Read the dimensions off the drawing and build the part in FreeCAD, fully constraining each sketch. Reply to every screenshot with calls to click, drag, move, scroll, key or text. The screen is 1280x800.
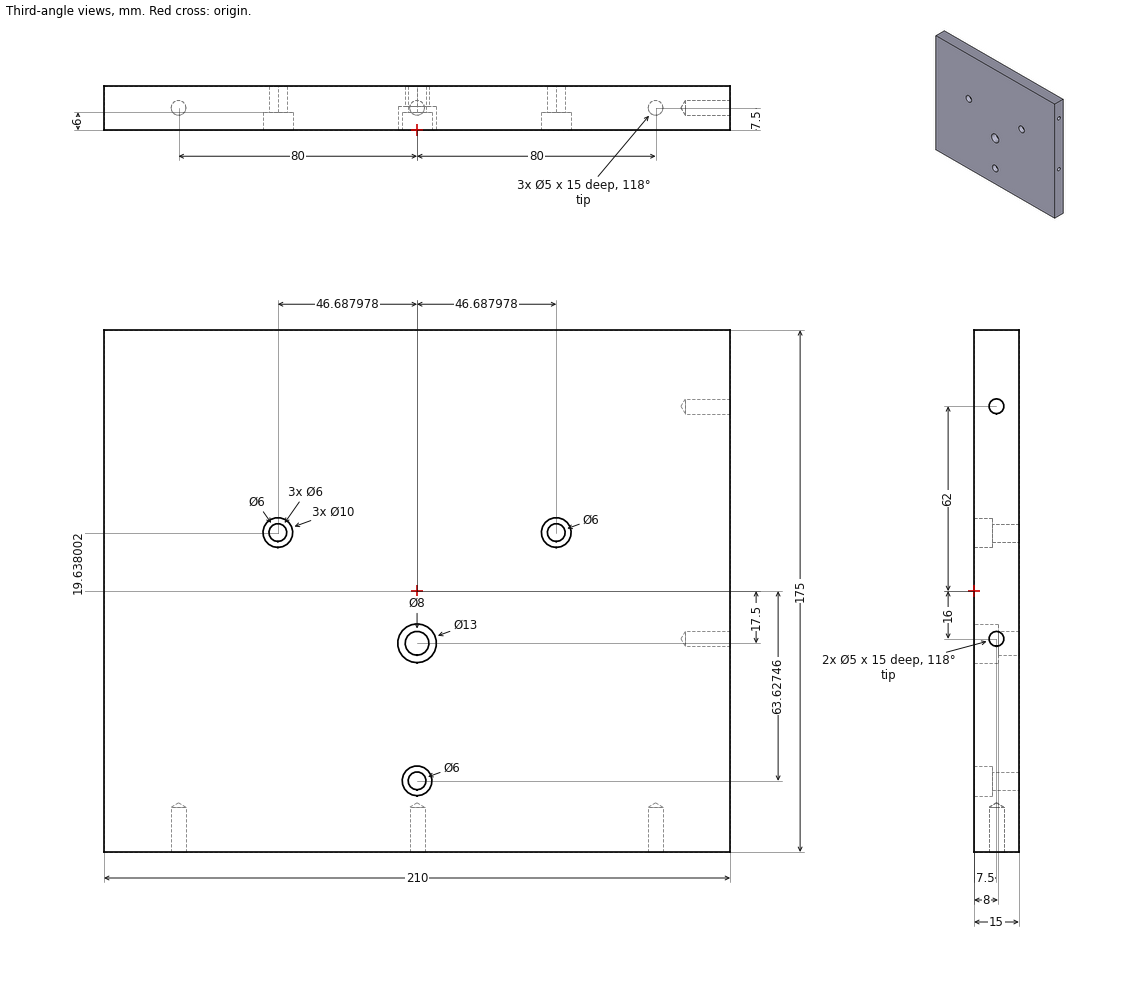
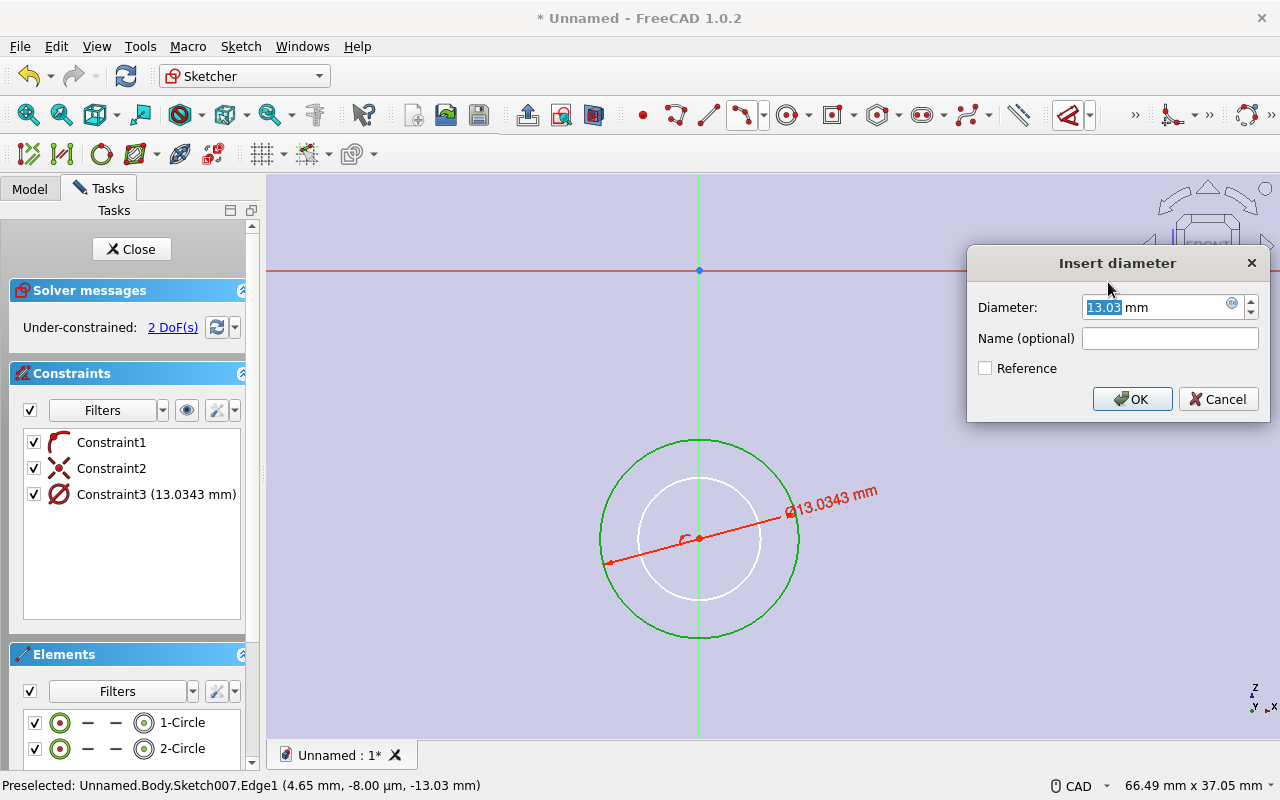
text(13)
key(Return)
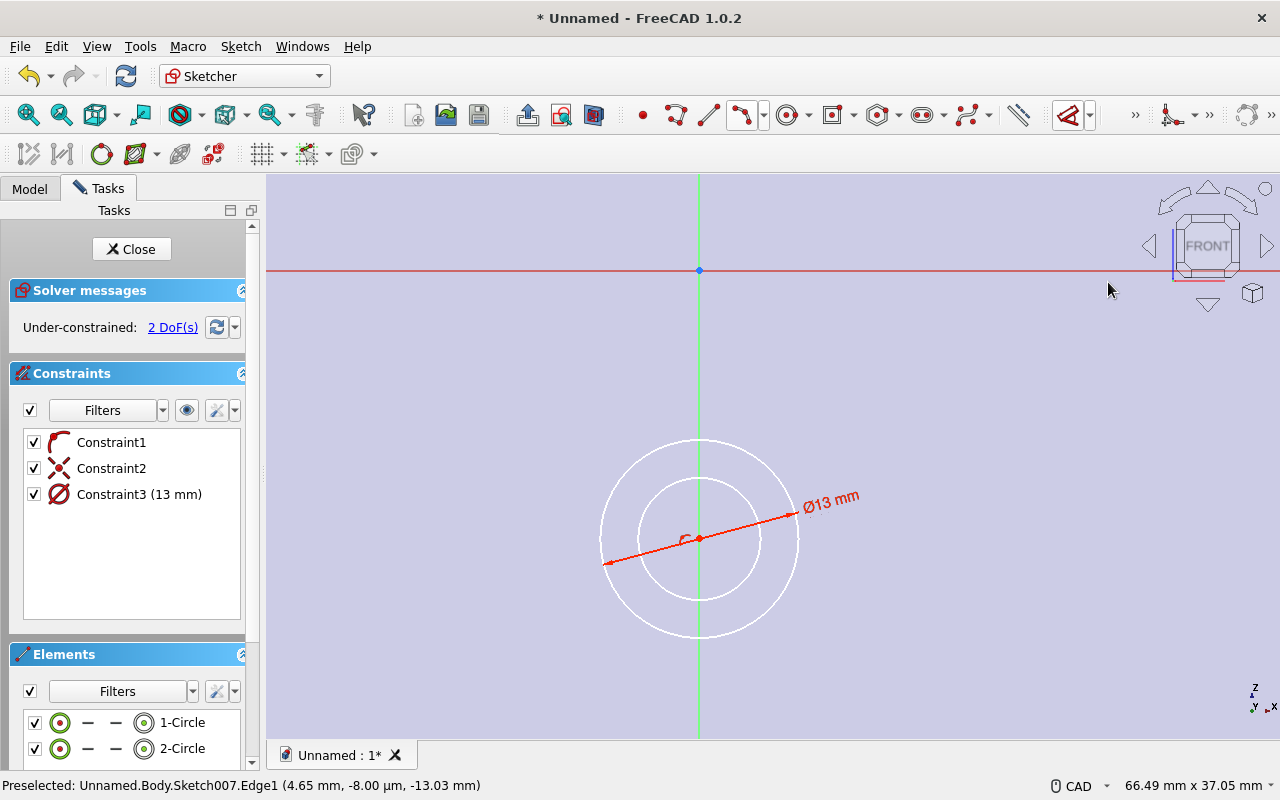
click(743, 496)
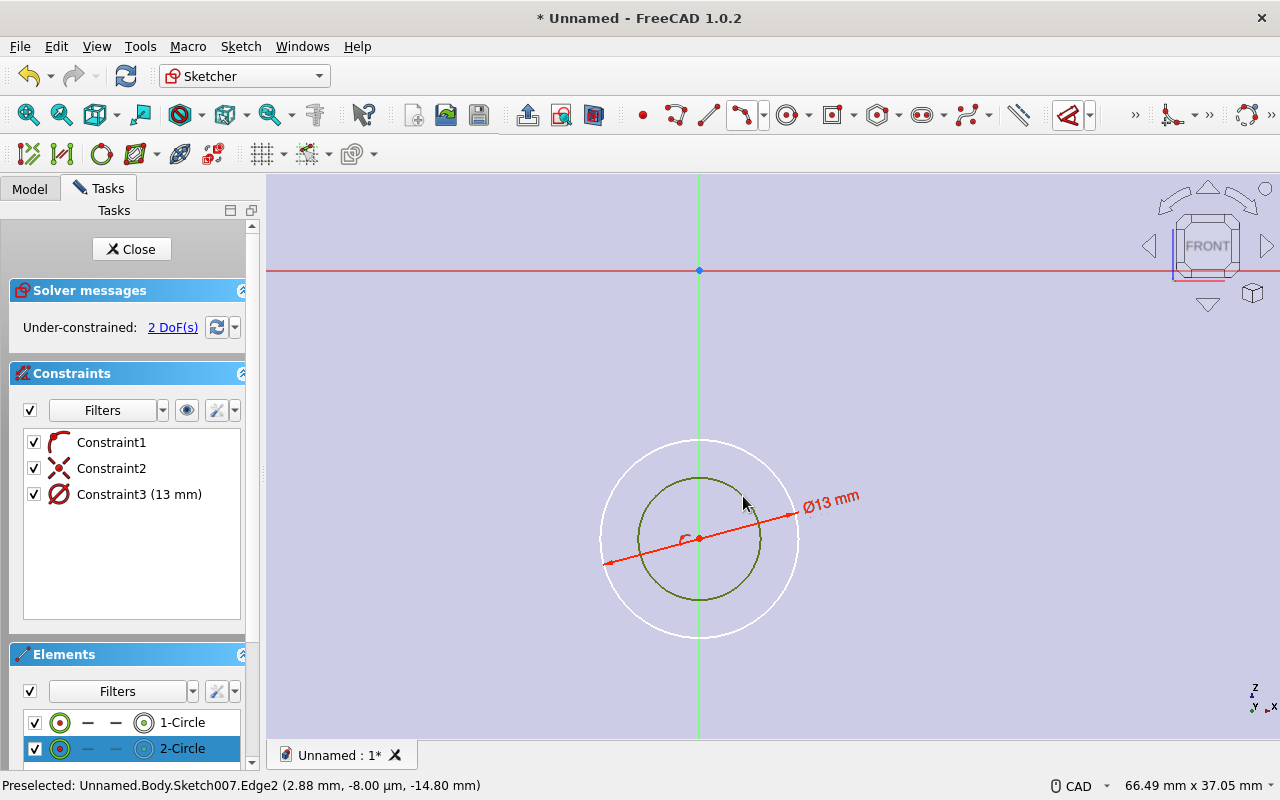
click(1090, 116)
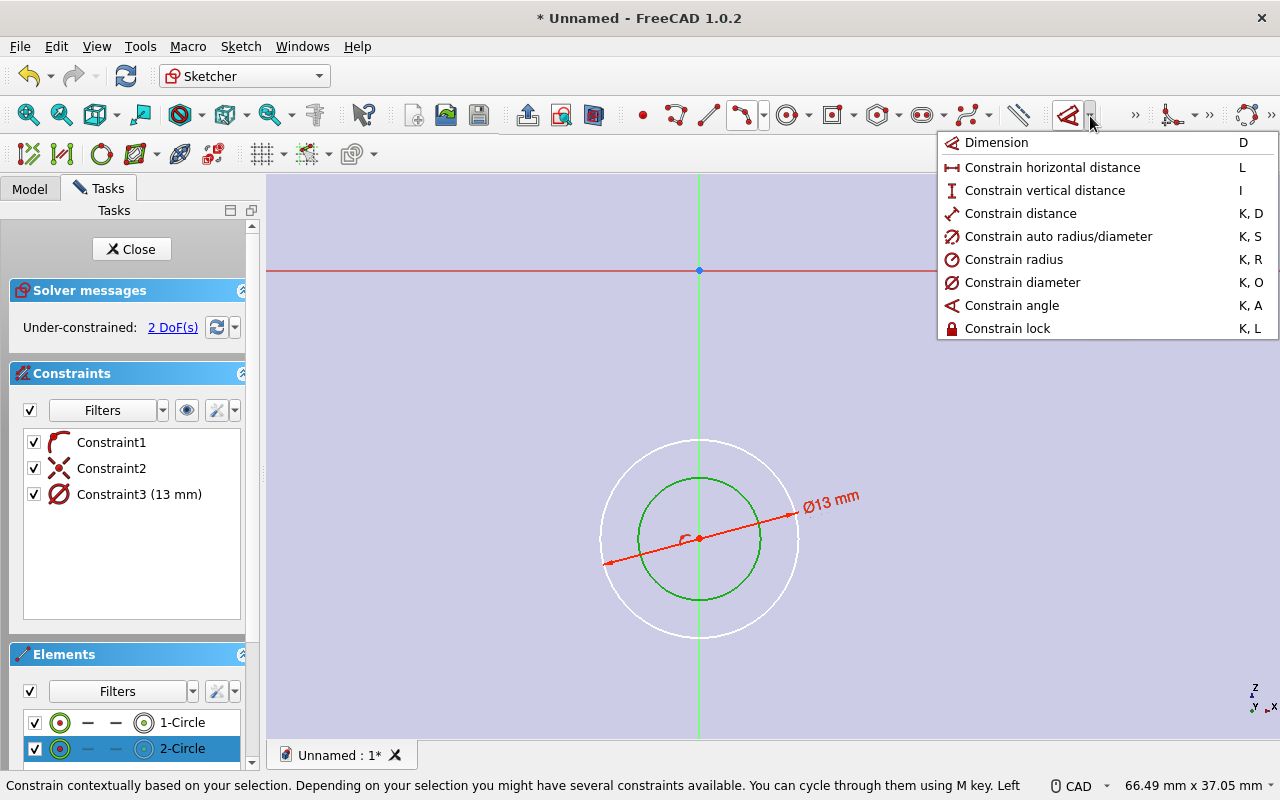
click(1108, 282)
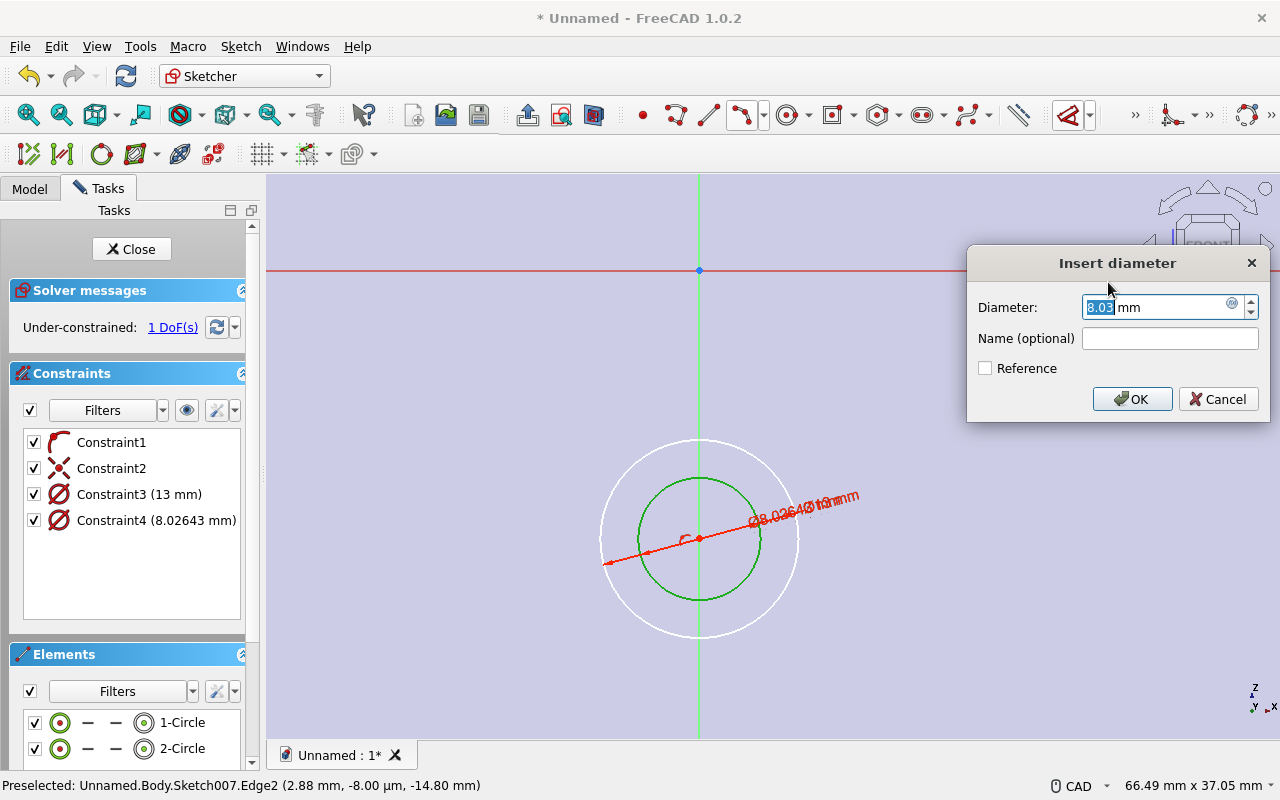
text(8)
key(Return)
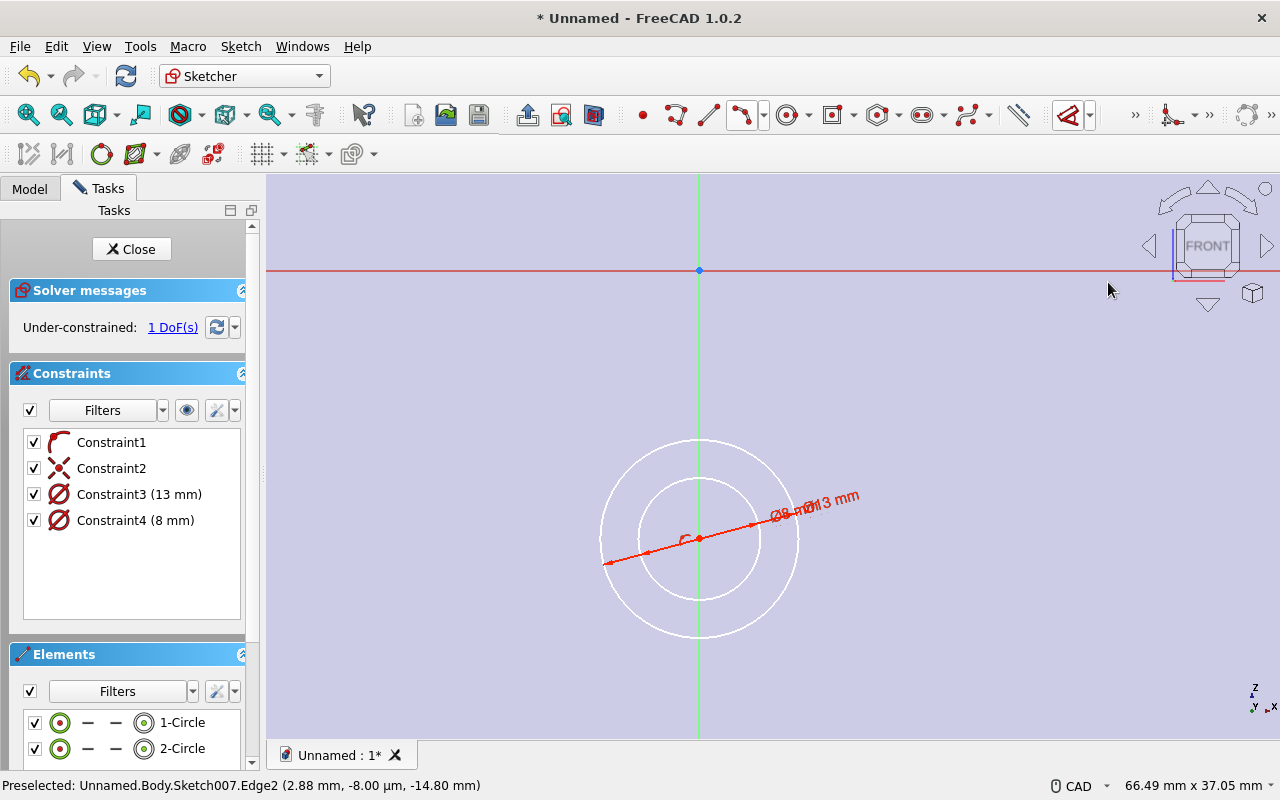
click(699, 539)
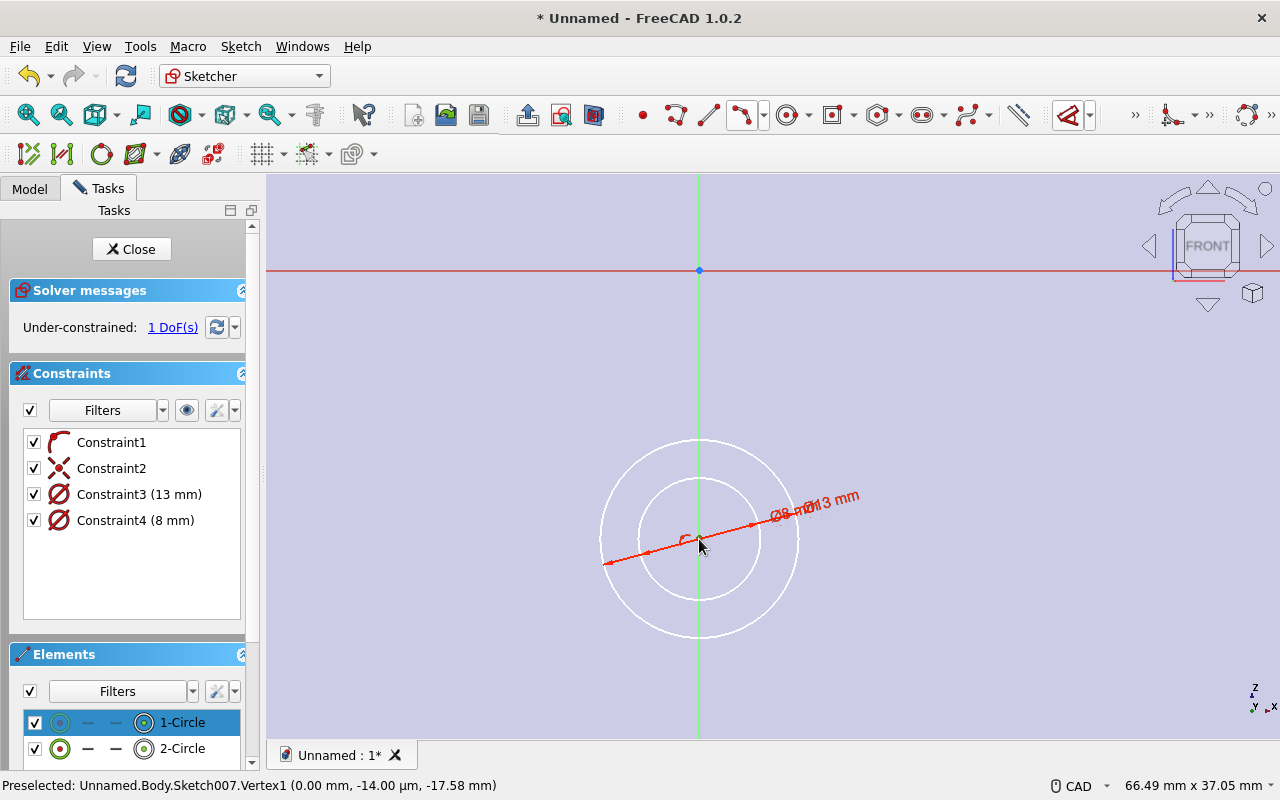
key(i)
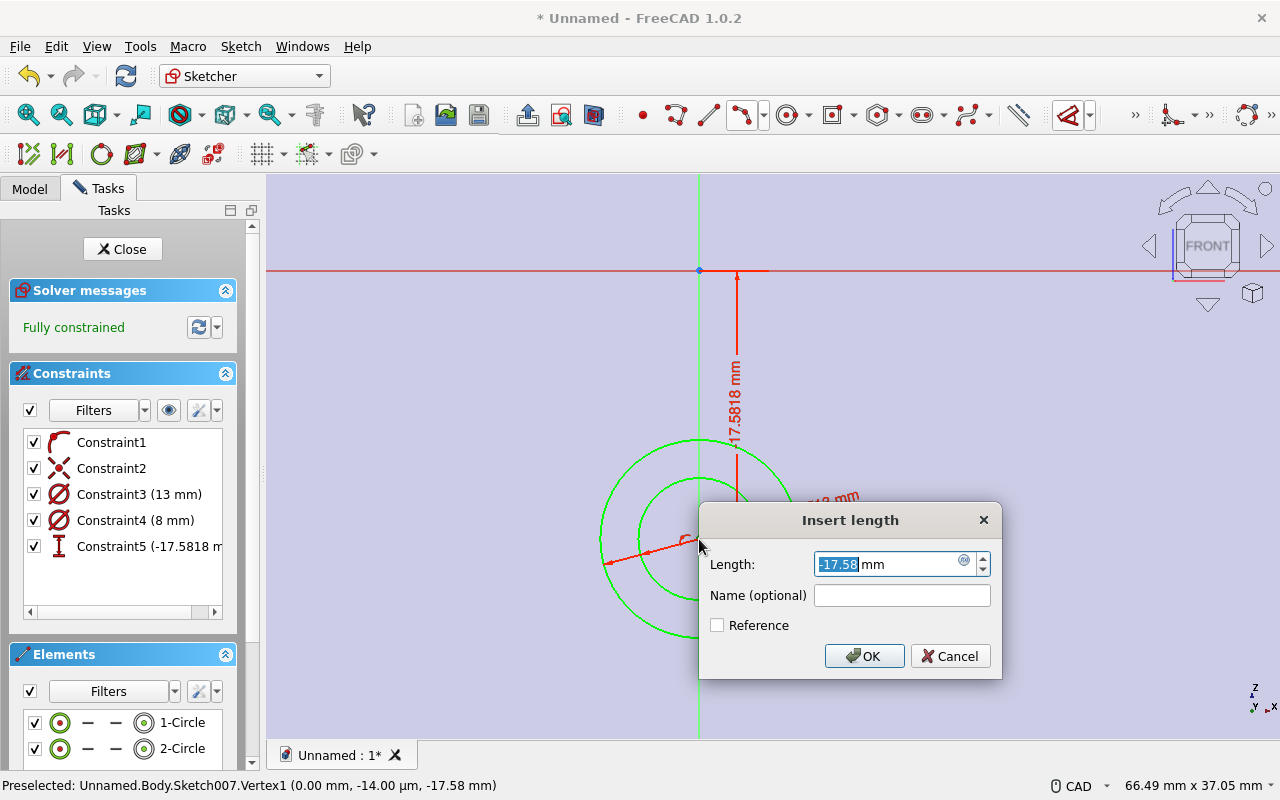
text(-17.5)
key(Return)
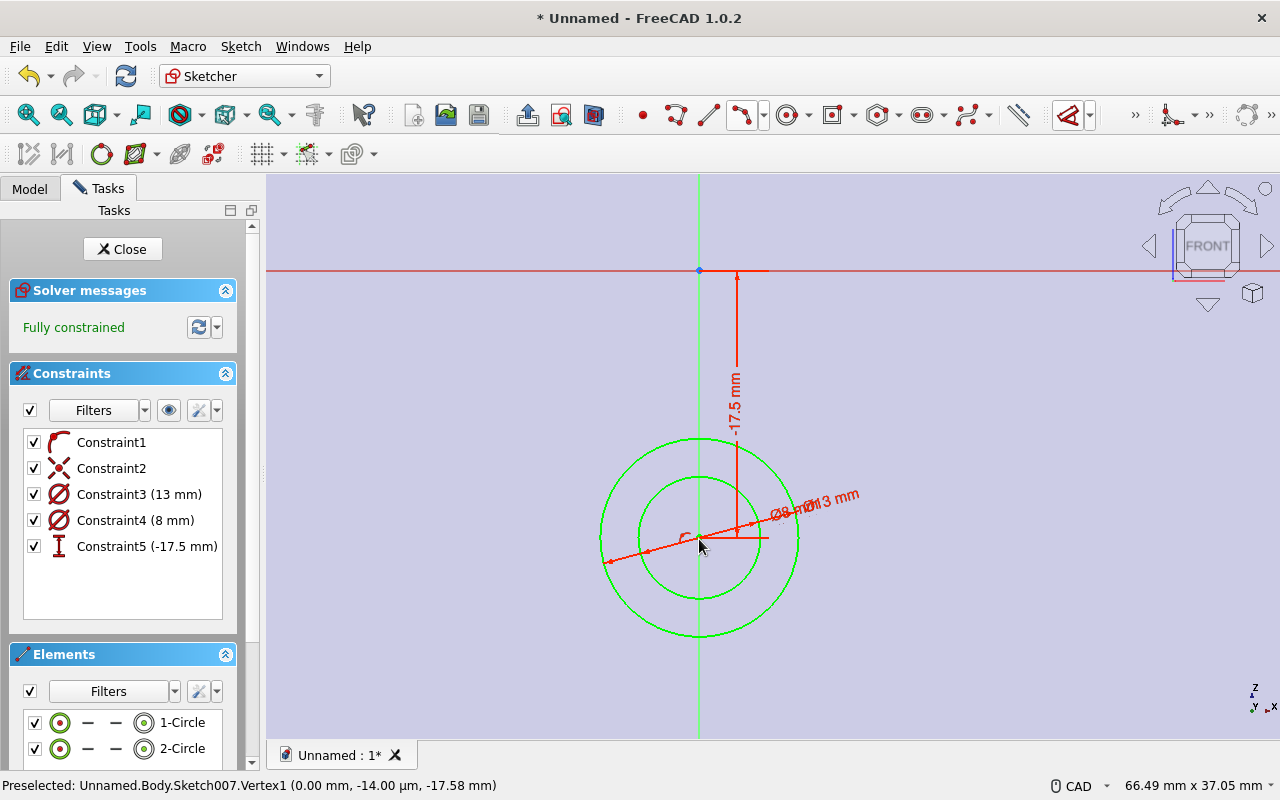
click(123, 249)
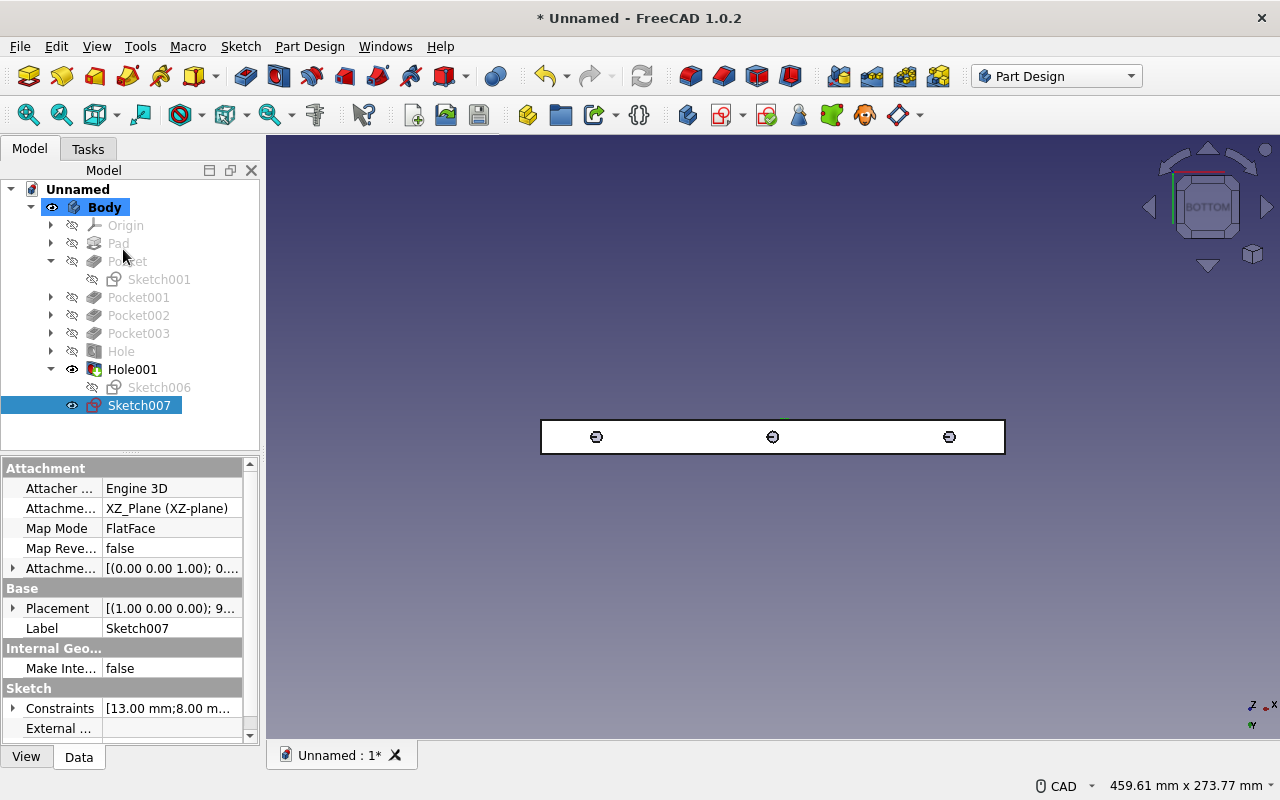
click(246, 76)